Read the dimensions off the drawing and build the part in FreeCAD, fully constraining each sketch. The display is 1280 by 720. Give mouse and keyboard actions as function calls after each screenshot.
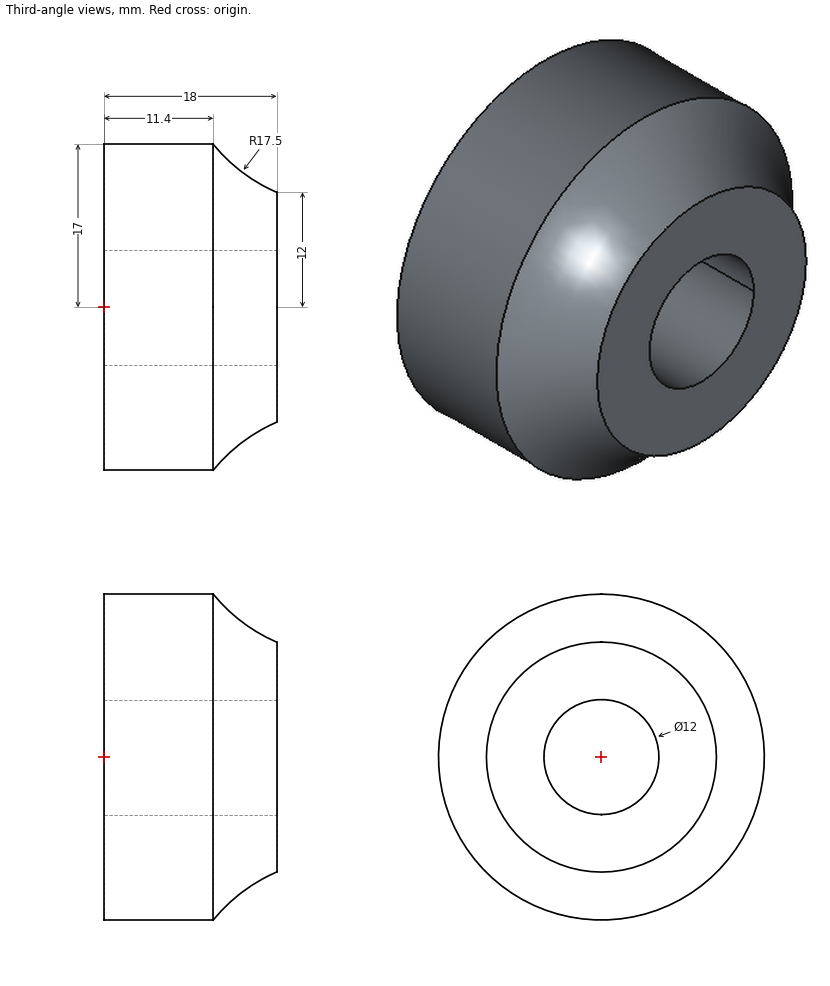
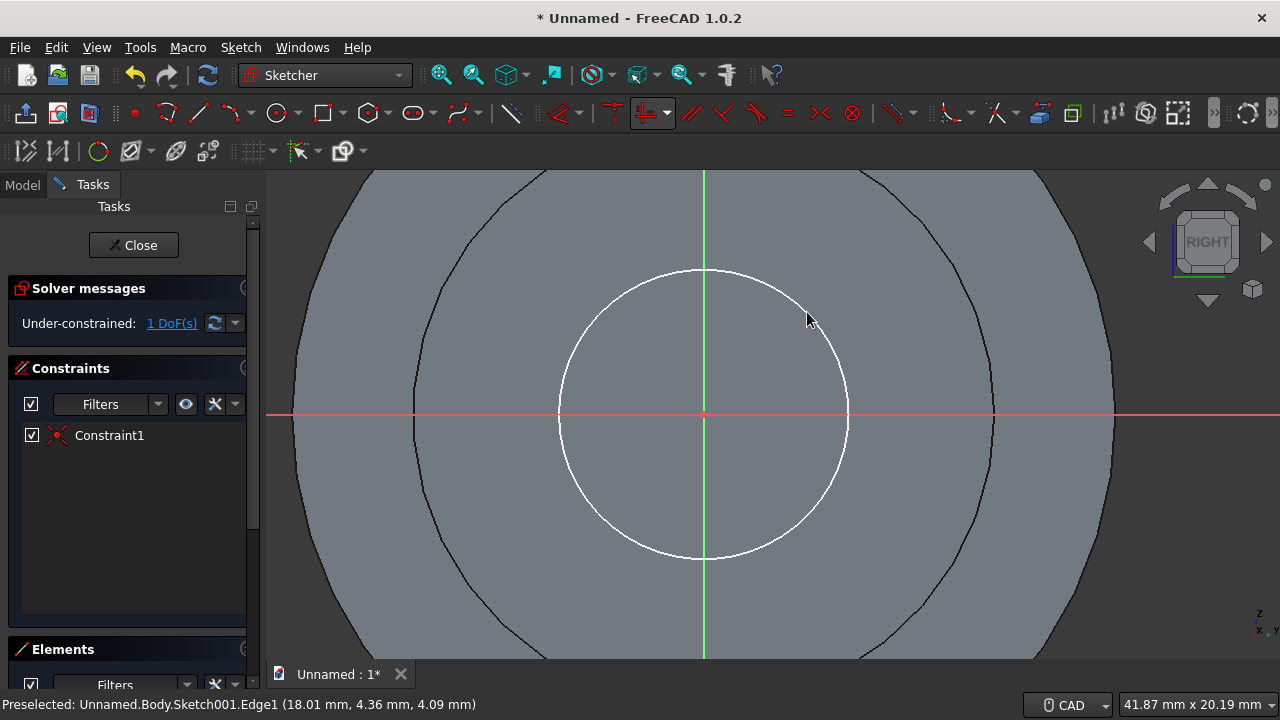
click(558, 114)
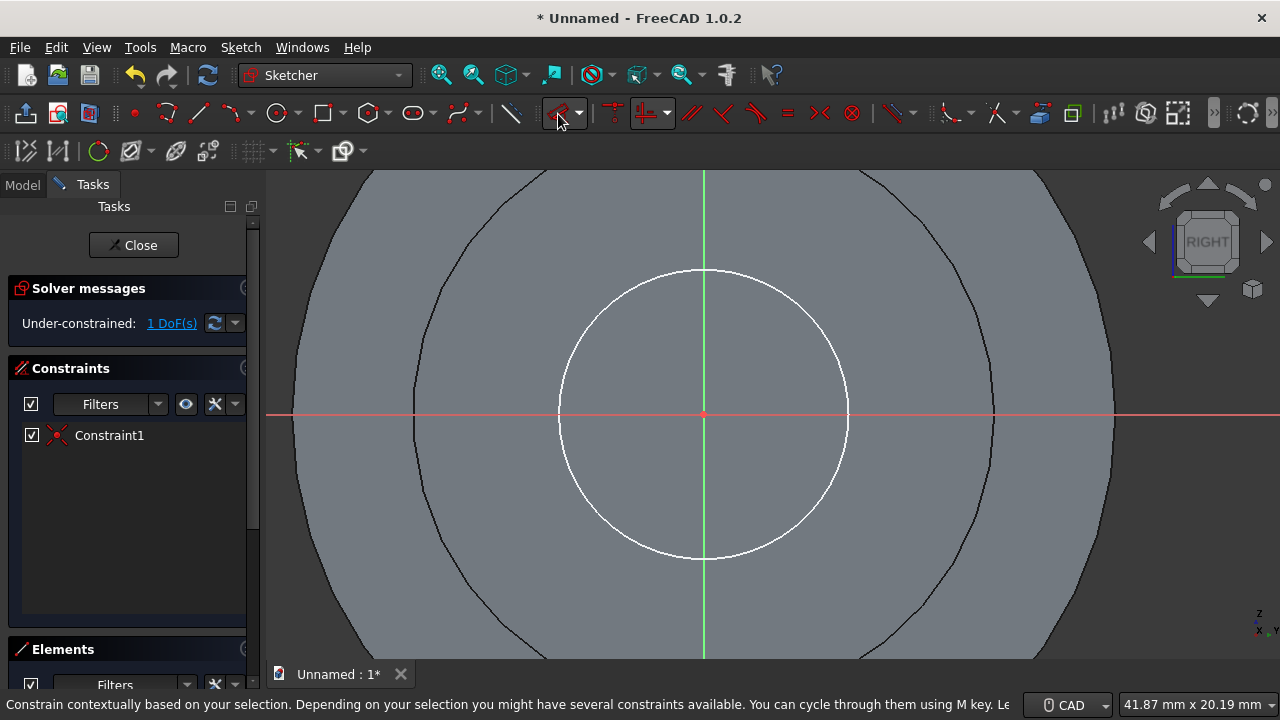
click(806, 312)
click(829, 289)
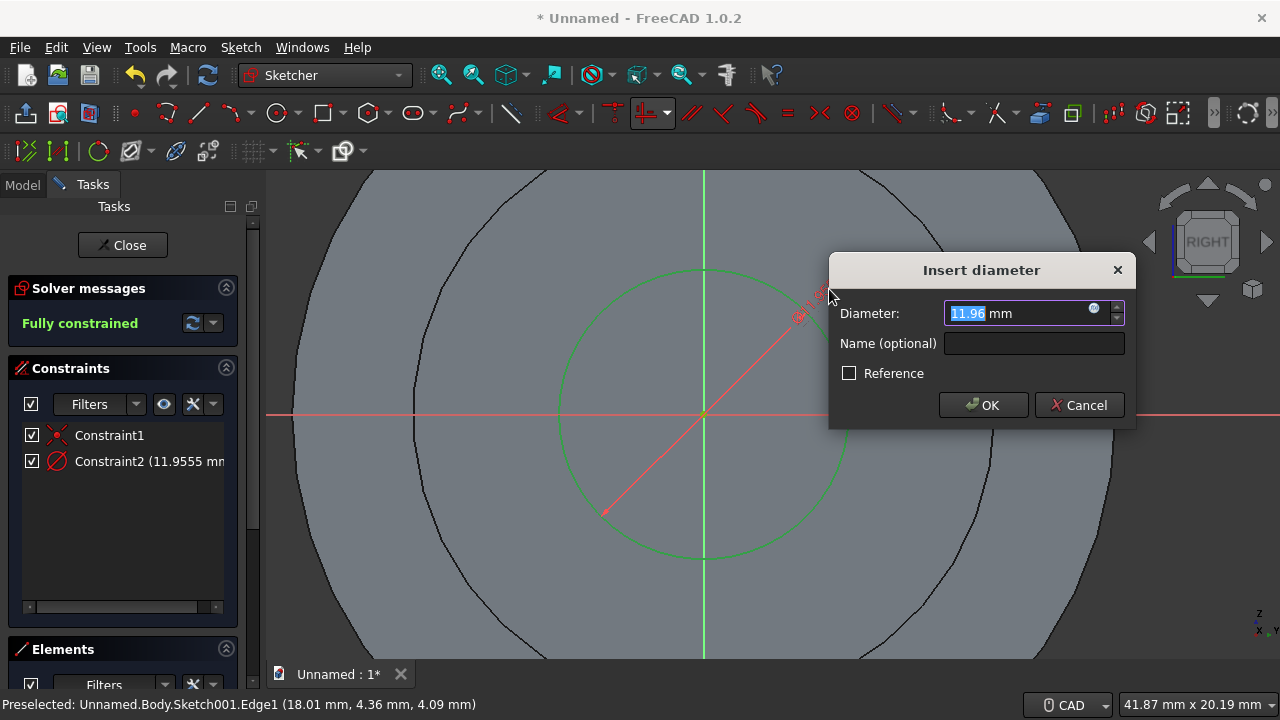
text(12)
key(Return)
key(Escape)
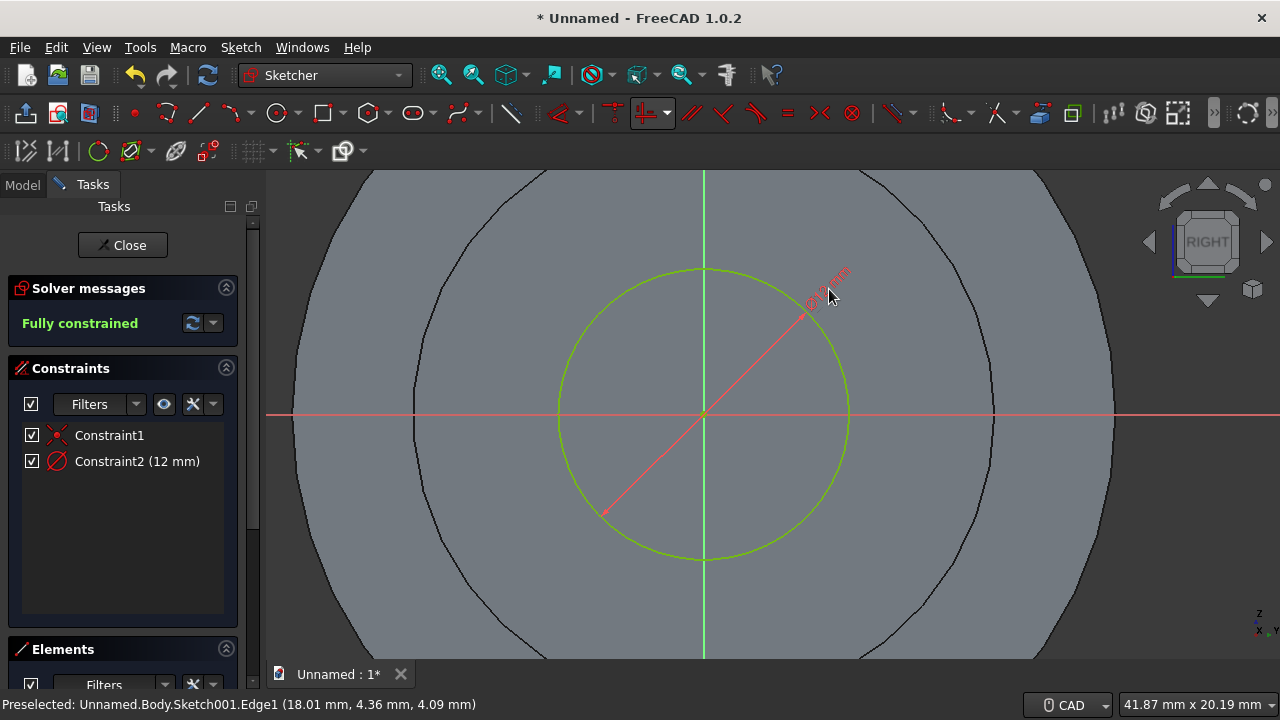
click(123, 245)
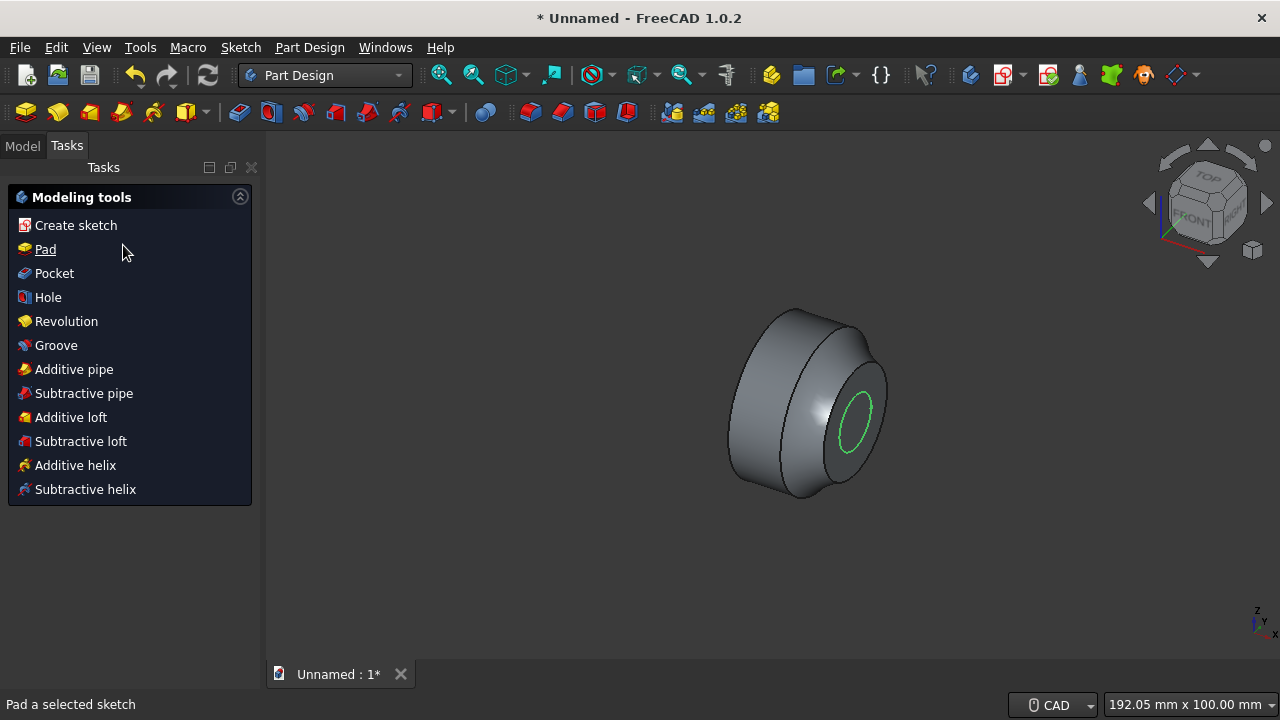
click(240, 112)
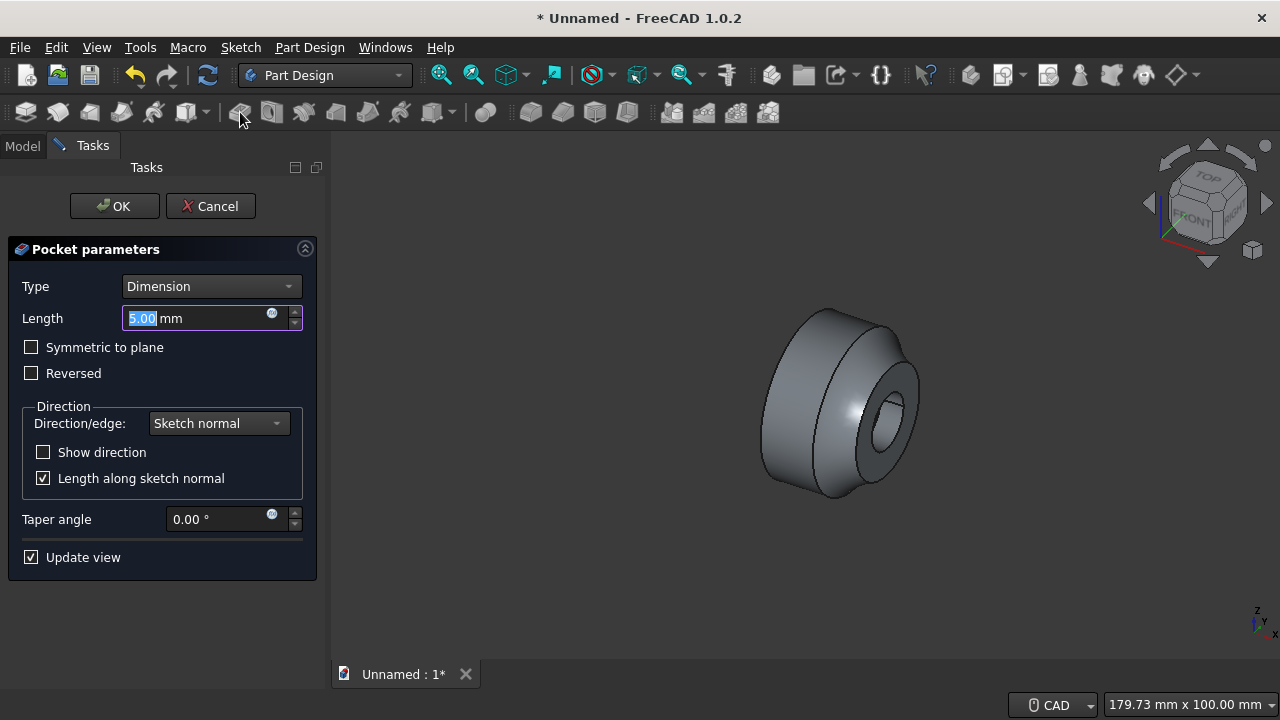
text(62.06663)
key(Tab)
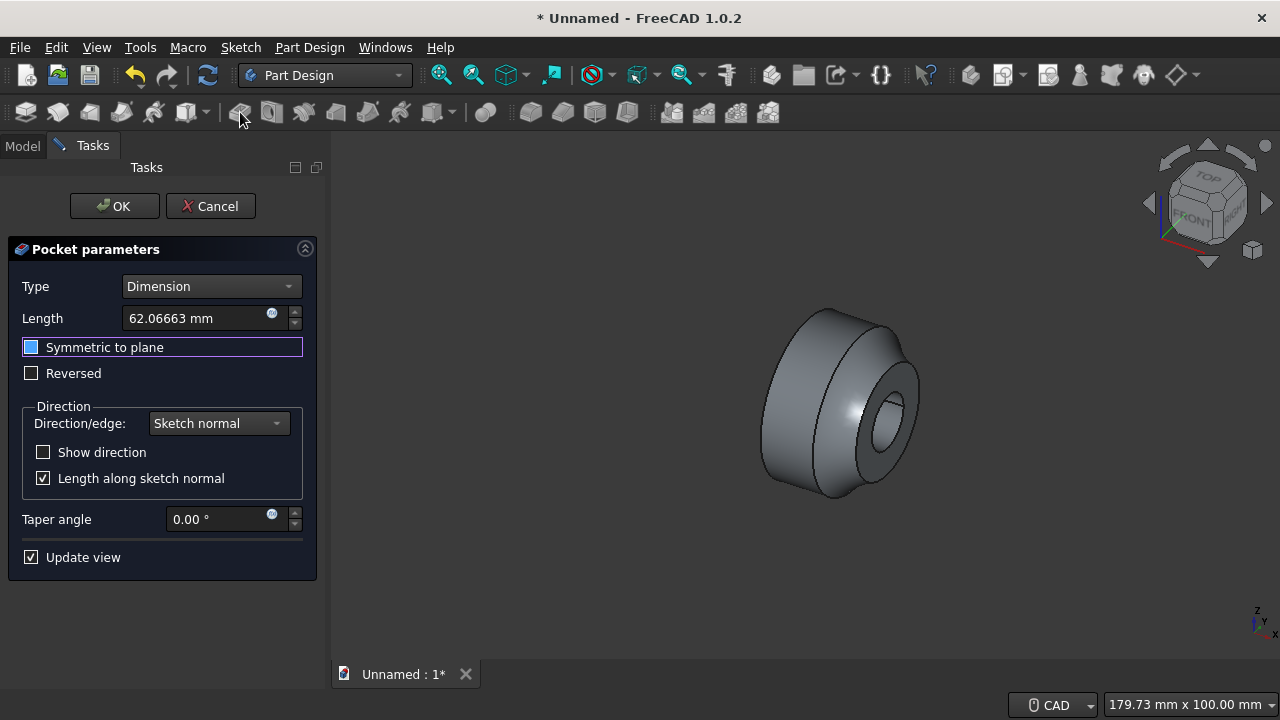
click(30, 347)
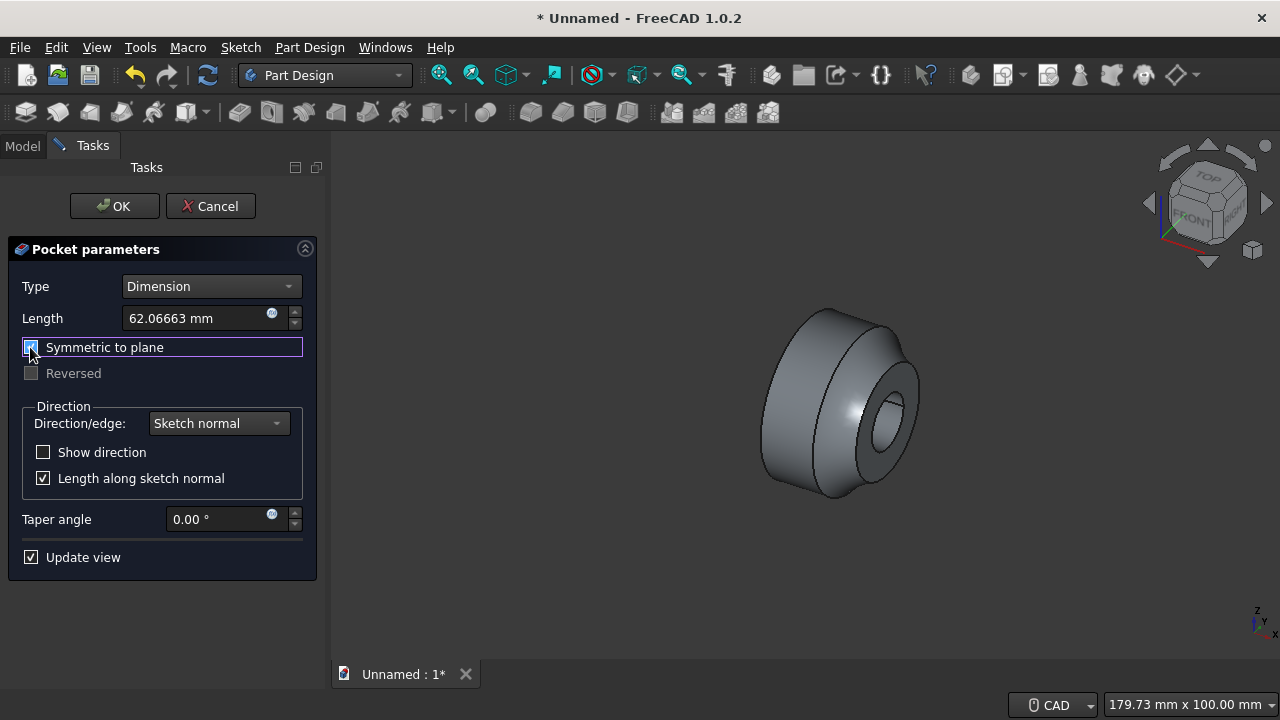
click(115, 206)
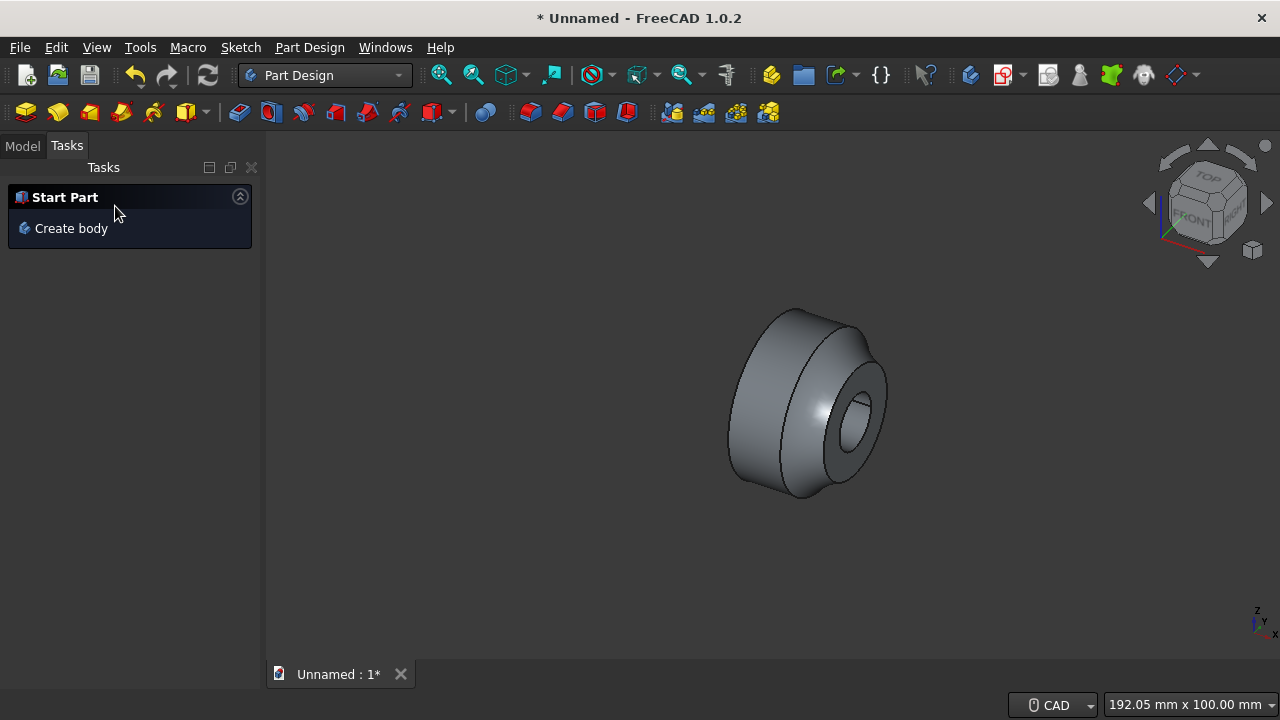
key(0)